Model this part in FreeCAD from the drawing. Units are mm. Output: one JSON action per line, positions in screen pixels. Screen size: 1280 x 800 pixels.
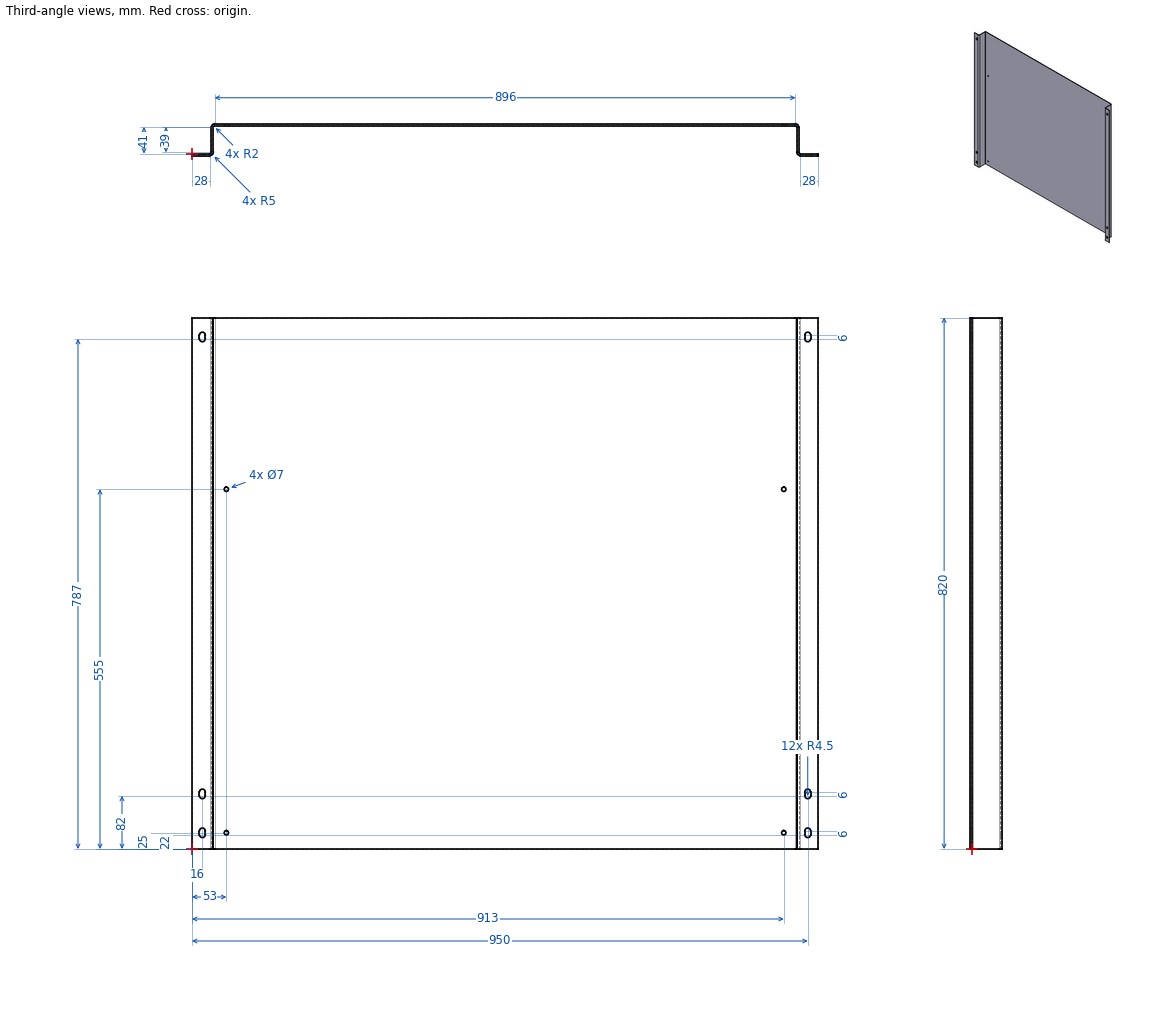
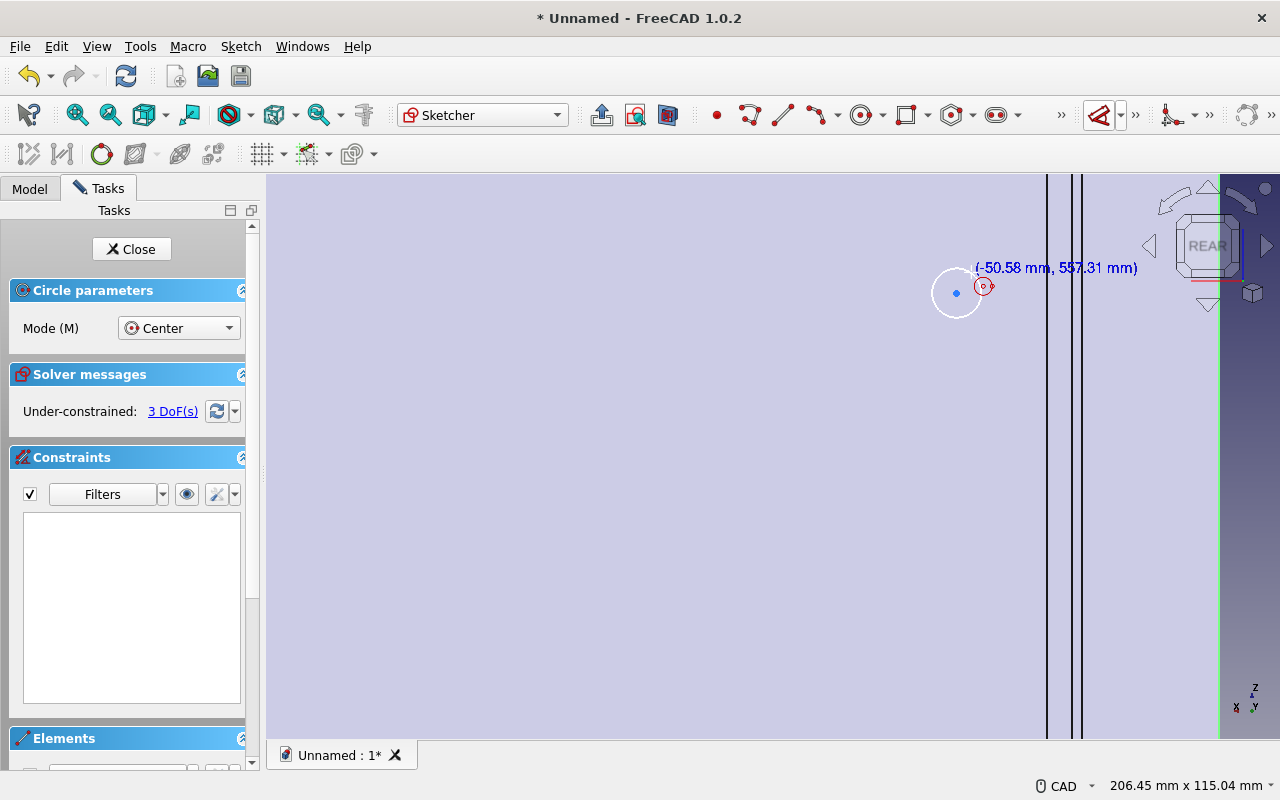
{"action": "scroll", "coordinate": [976, 271], "scroll_direction": "down", "scroll_amount": 10}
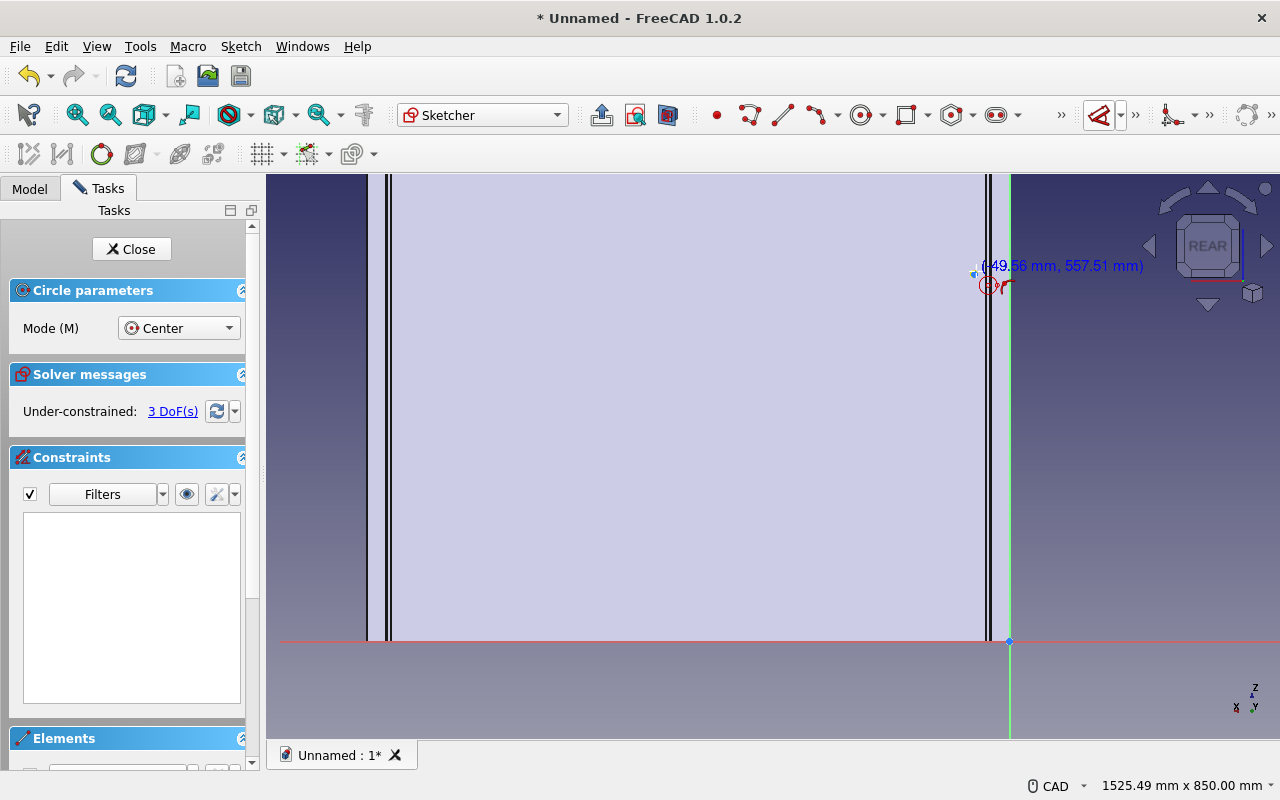
{"action": "scroll", "coordinate": [974, 625], "scroll_direction": "up", "scroll_amount": 12}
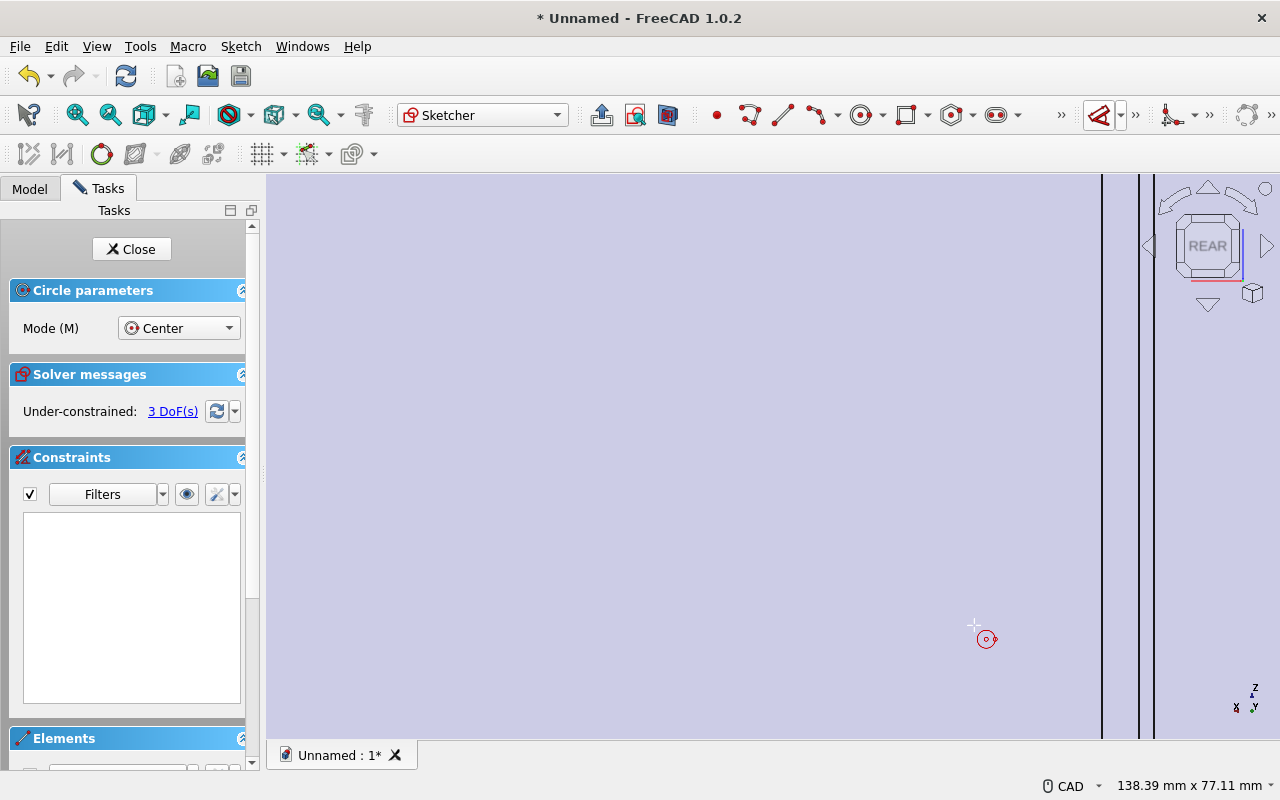
{"action": "scroll", "coordinate": [974, 626], "scroll_direction": "down", "scroll_amount": 12}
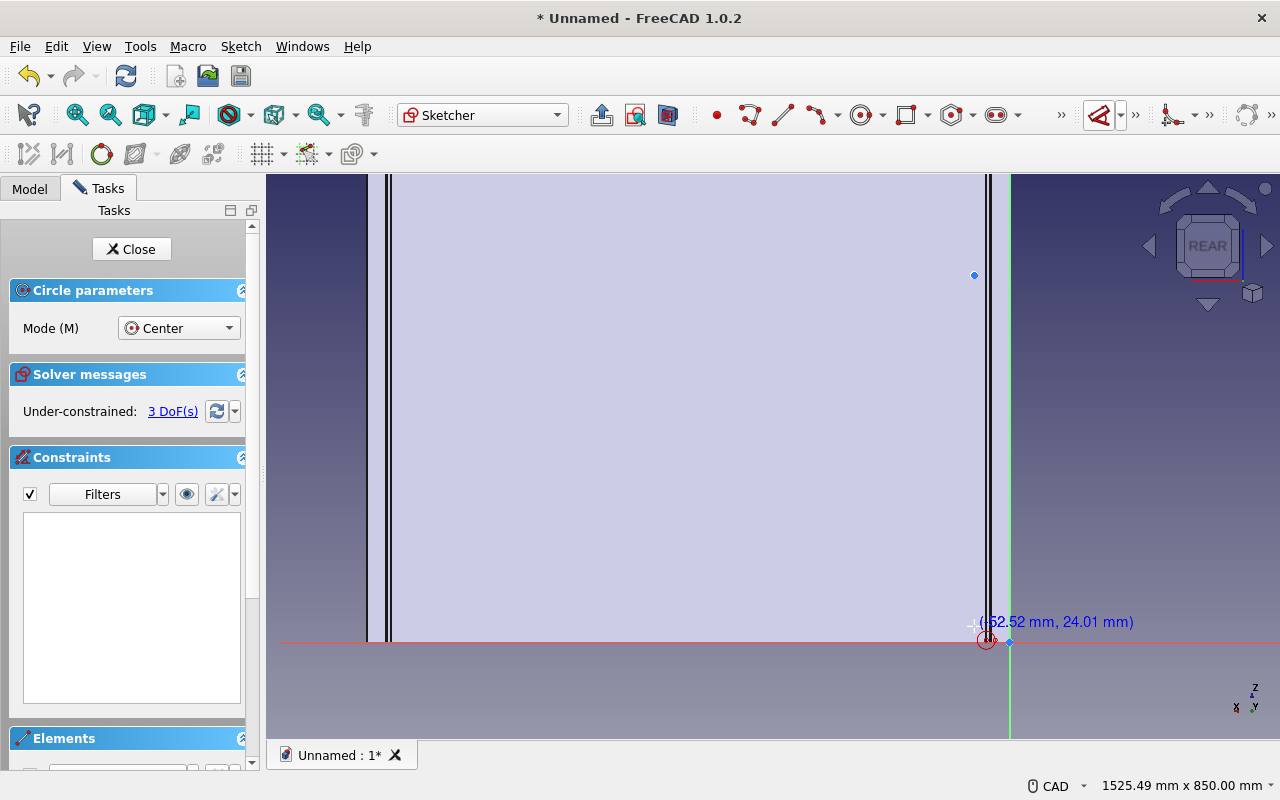
{"action": "left_click", "coordinate": [974, 626]}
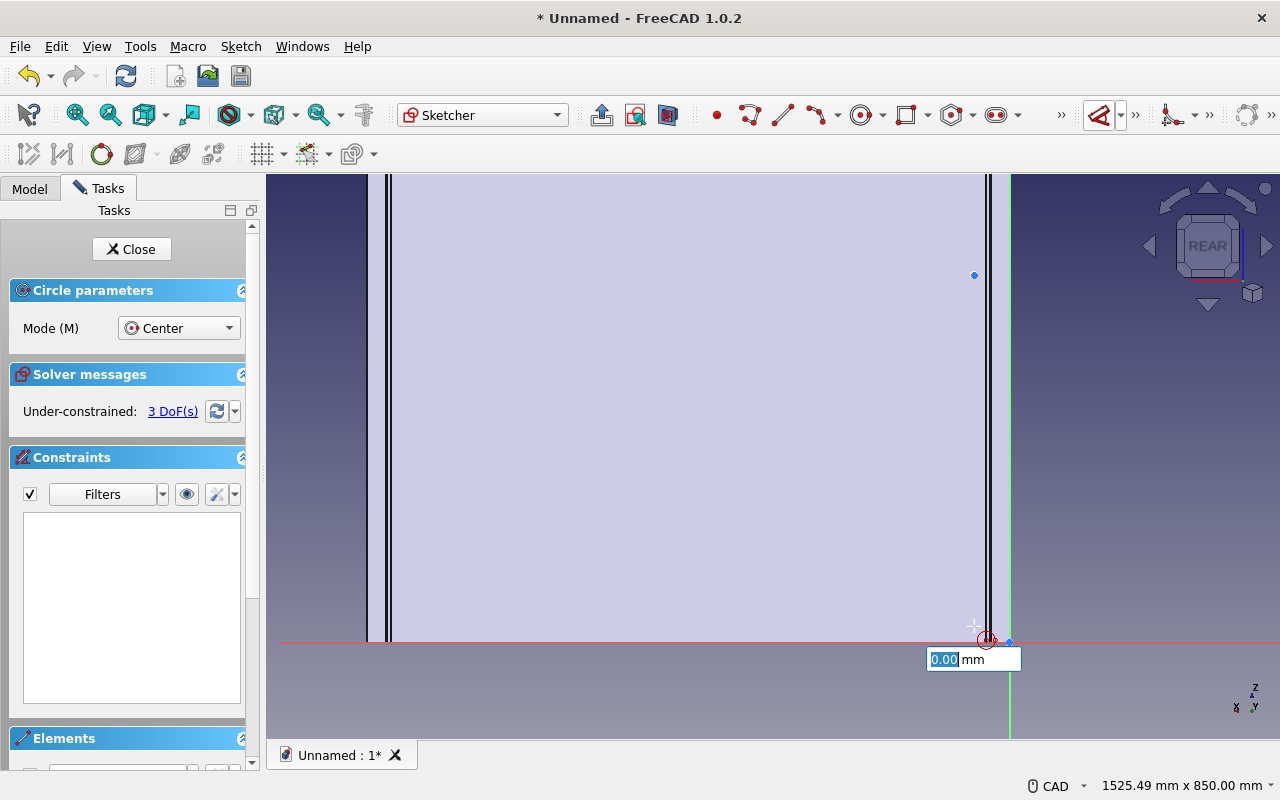
{"action": "scroll", "coordinate": [976, 625], "scroll_direction": "up", "scroll_amount": 10}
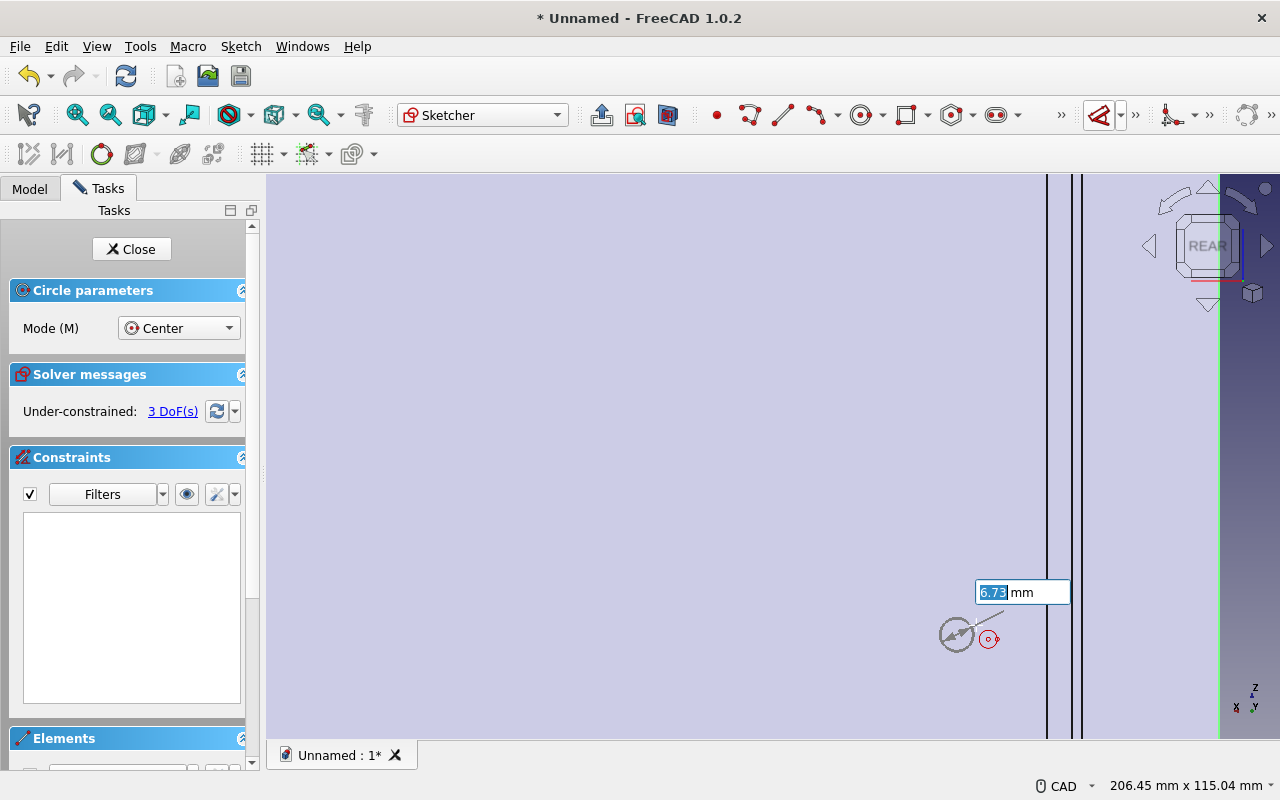
{"action": "left_click", "coordinate": [971, 616]}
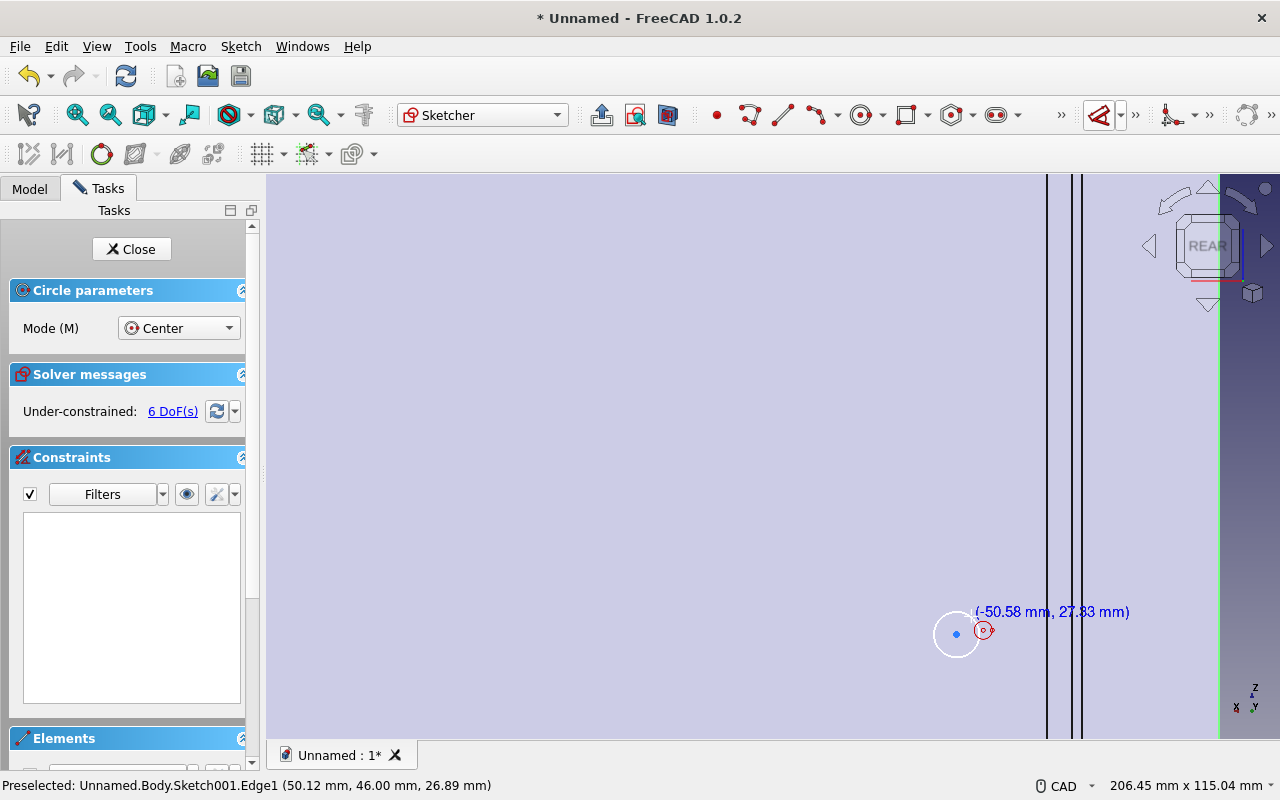
{"action": "scroll", "coordinate": [976, 625], "scroll_direction": "down", "scroll_amount": 10}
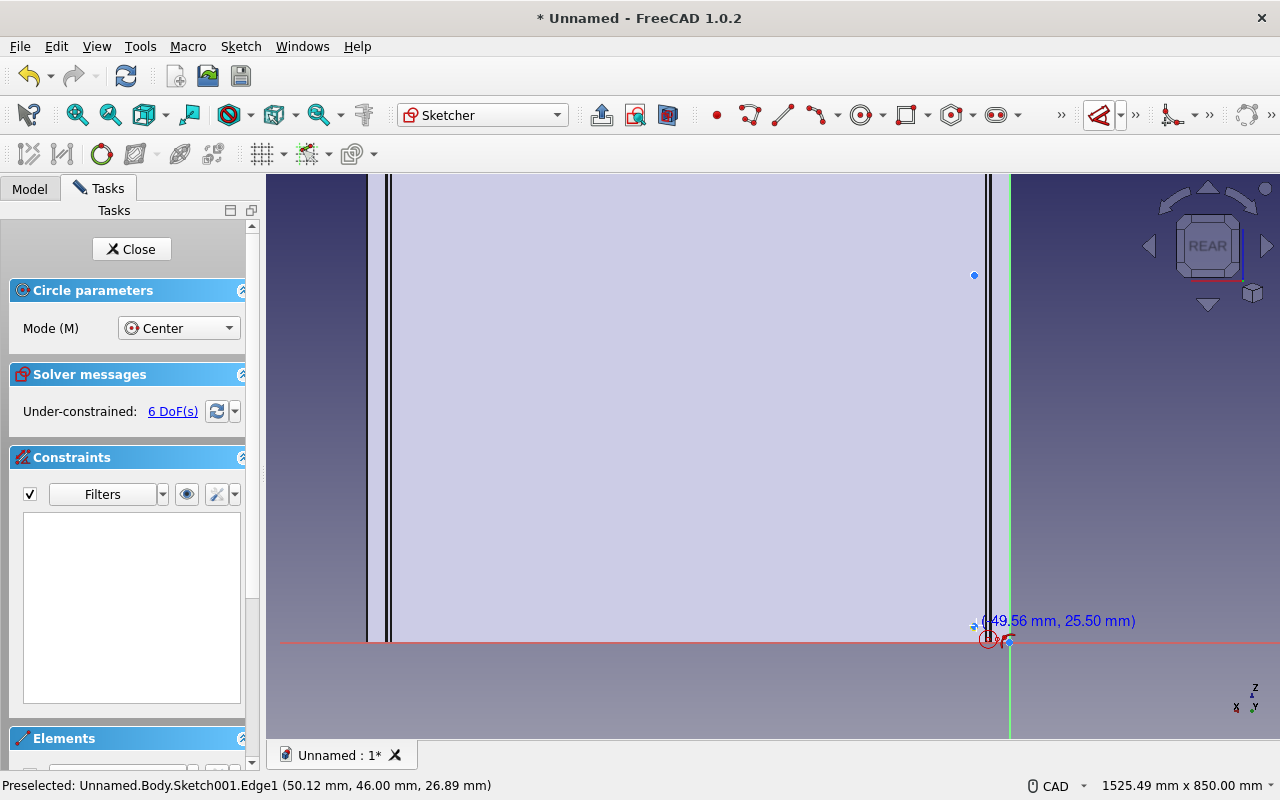
{"action": "scroll", "coordinate": [403, 626], "scroll_direction": "up", "scroll_amount": 12}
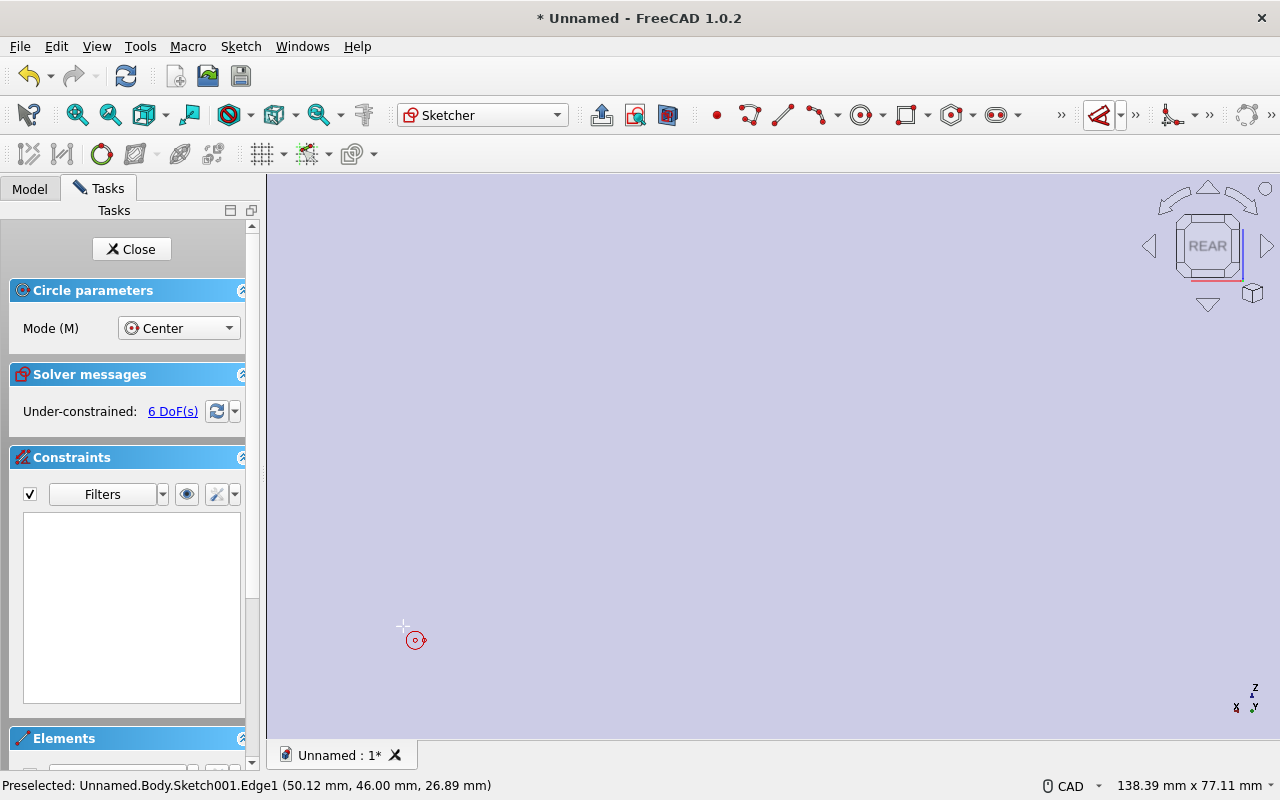
{"action": "scroll", "coordinate": [403, 626], "scroll_direction": "down", "scroll_amount": 12}